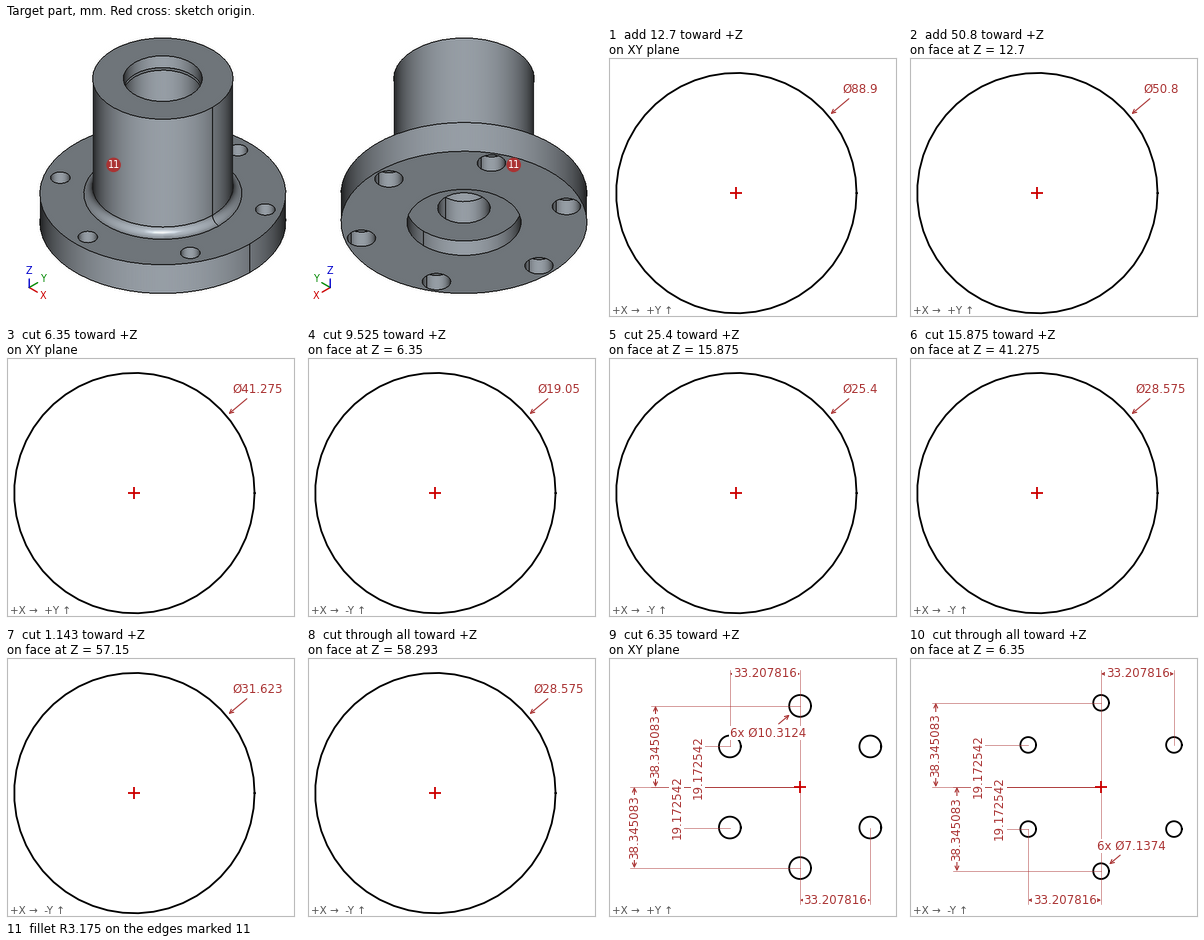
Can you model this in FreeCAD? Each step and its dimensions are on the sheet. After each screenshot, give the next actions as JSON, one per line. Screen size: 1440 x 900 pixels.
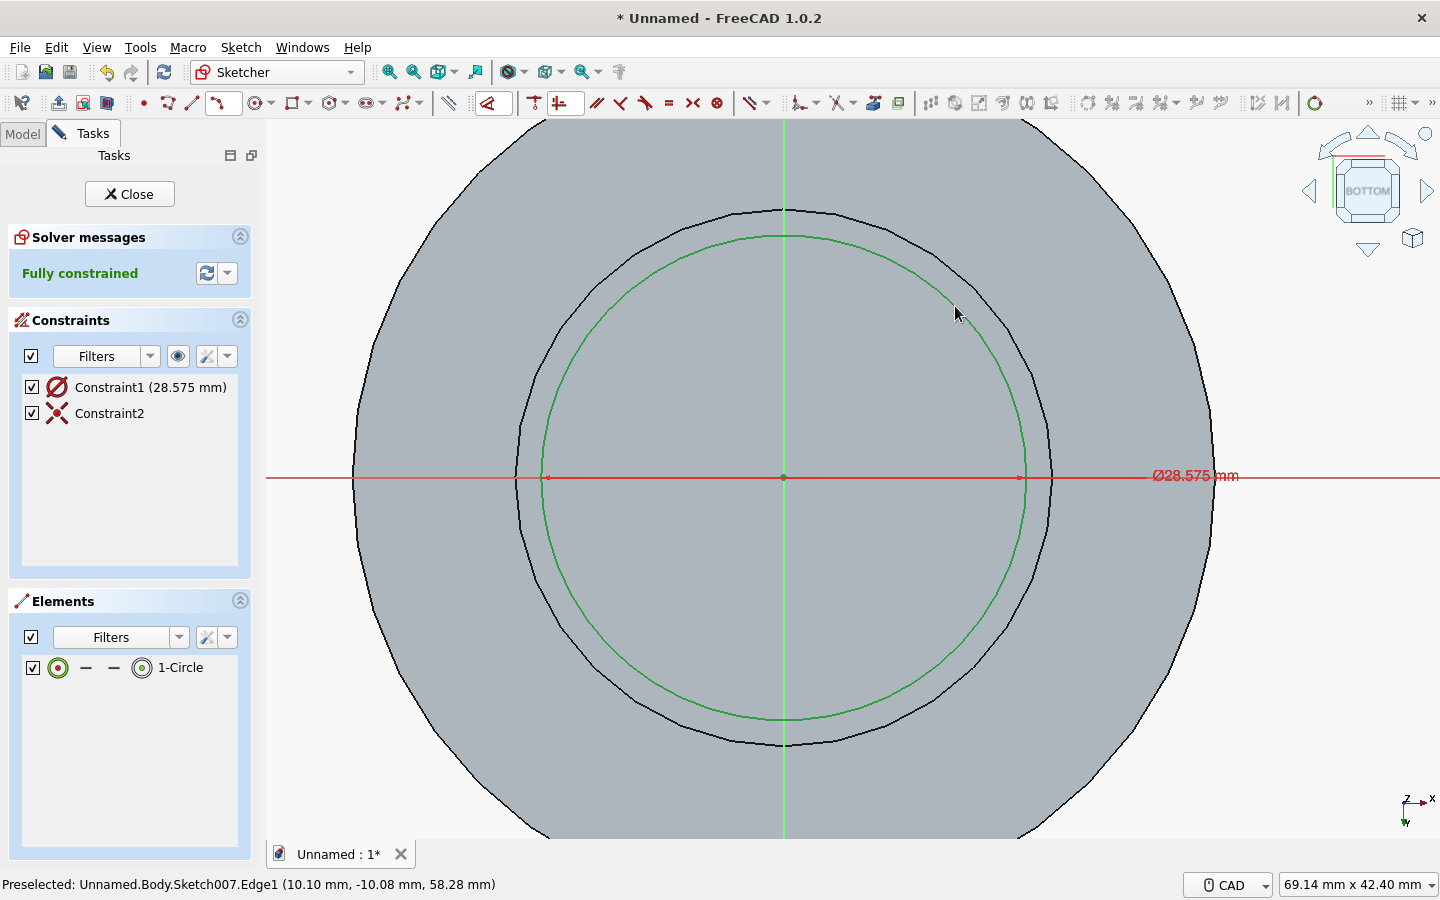
{"action": "left_click", "coordinate": [130, 194]}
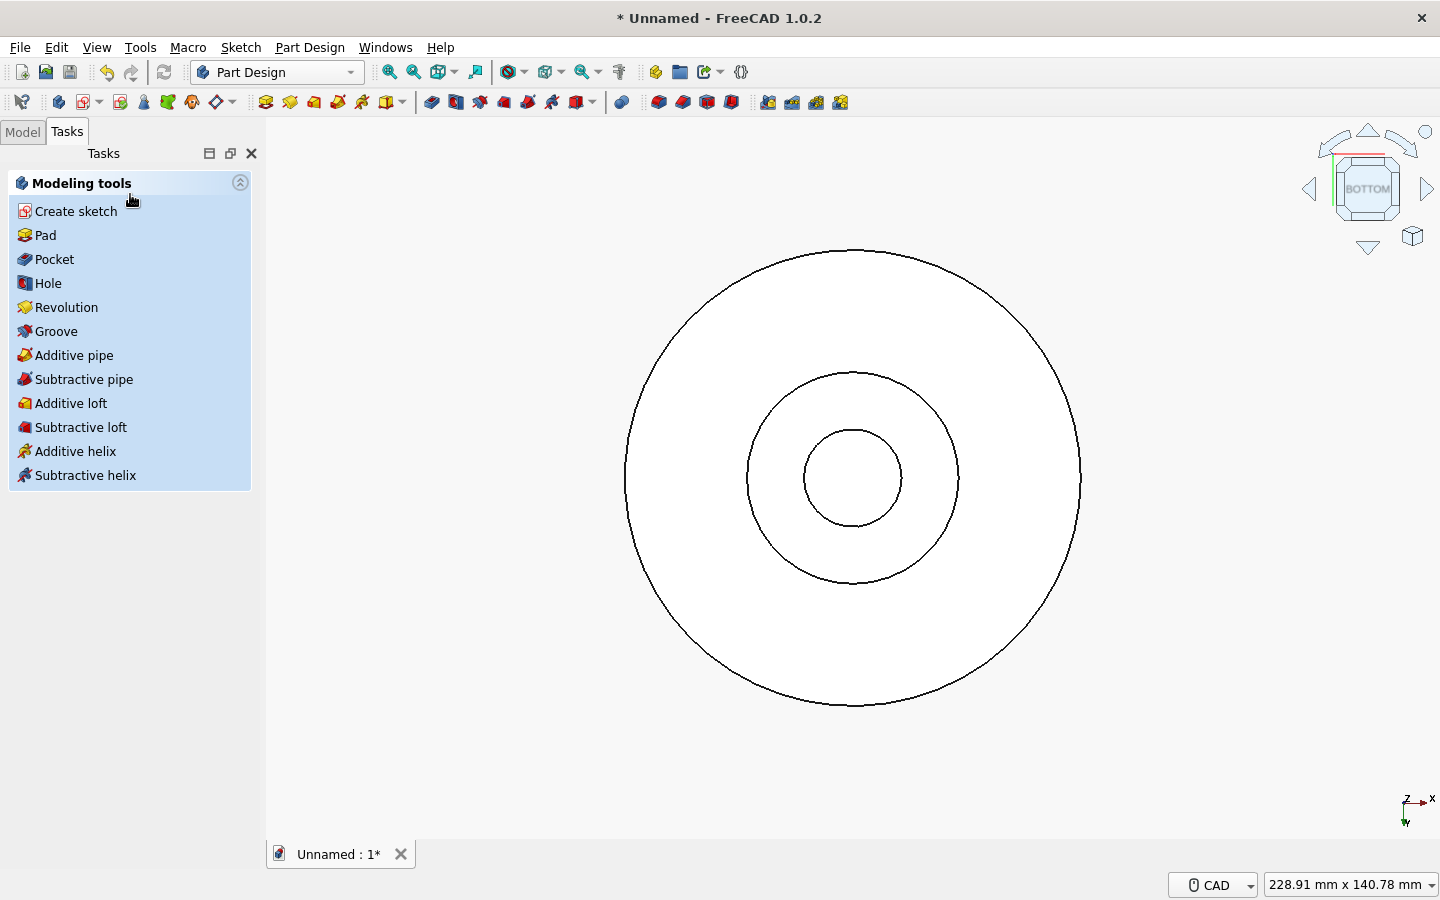
{"action": "left_click", "coordinate": [432, 102]}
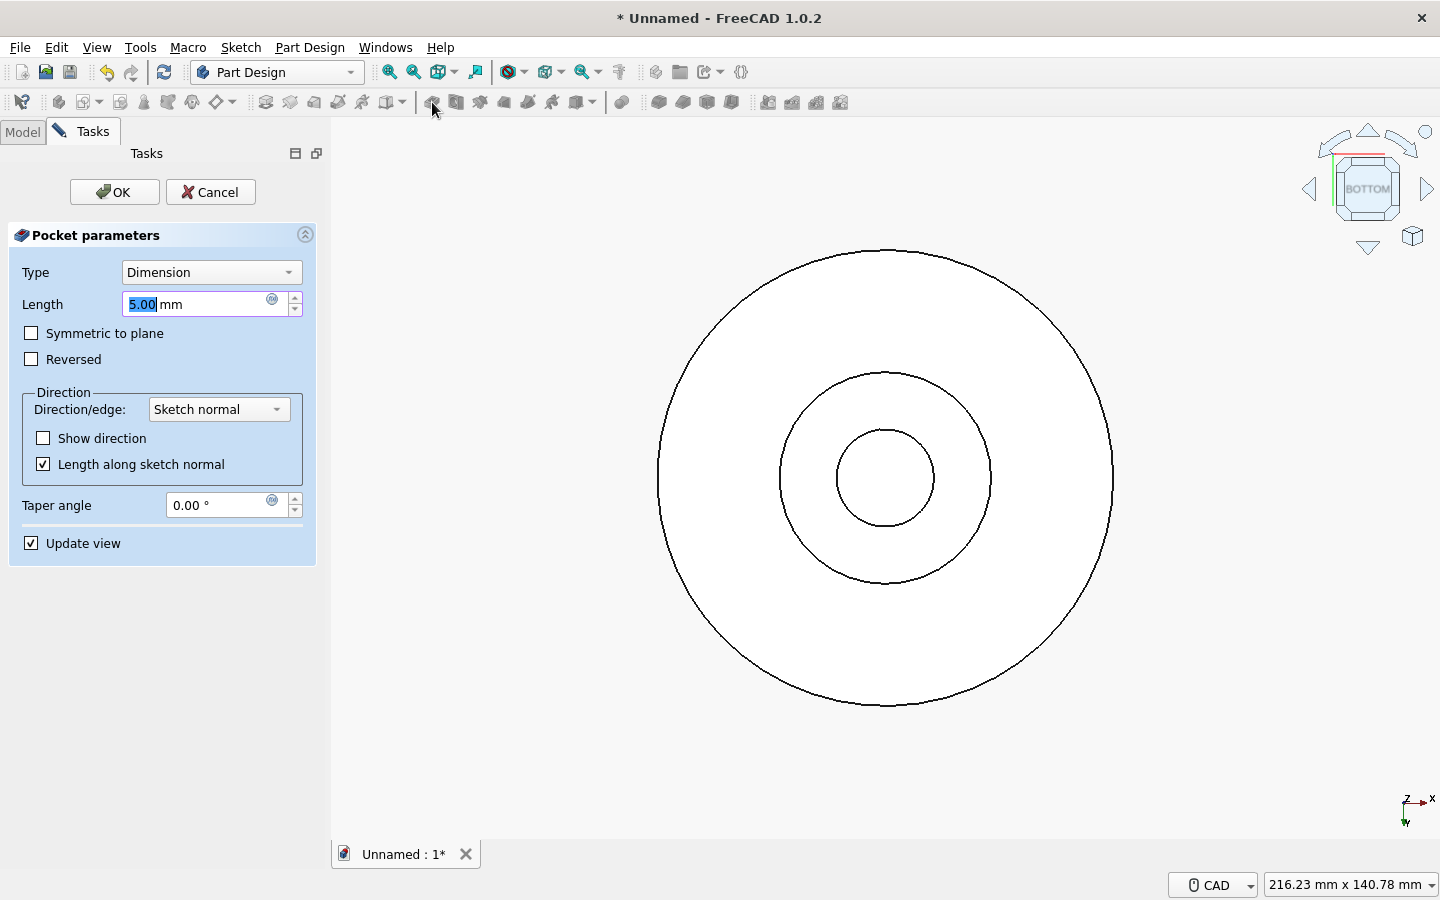
{"action": "left_click", "coordinate": [212, 272]}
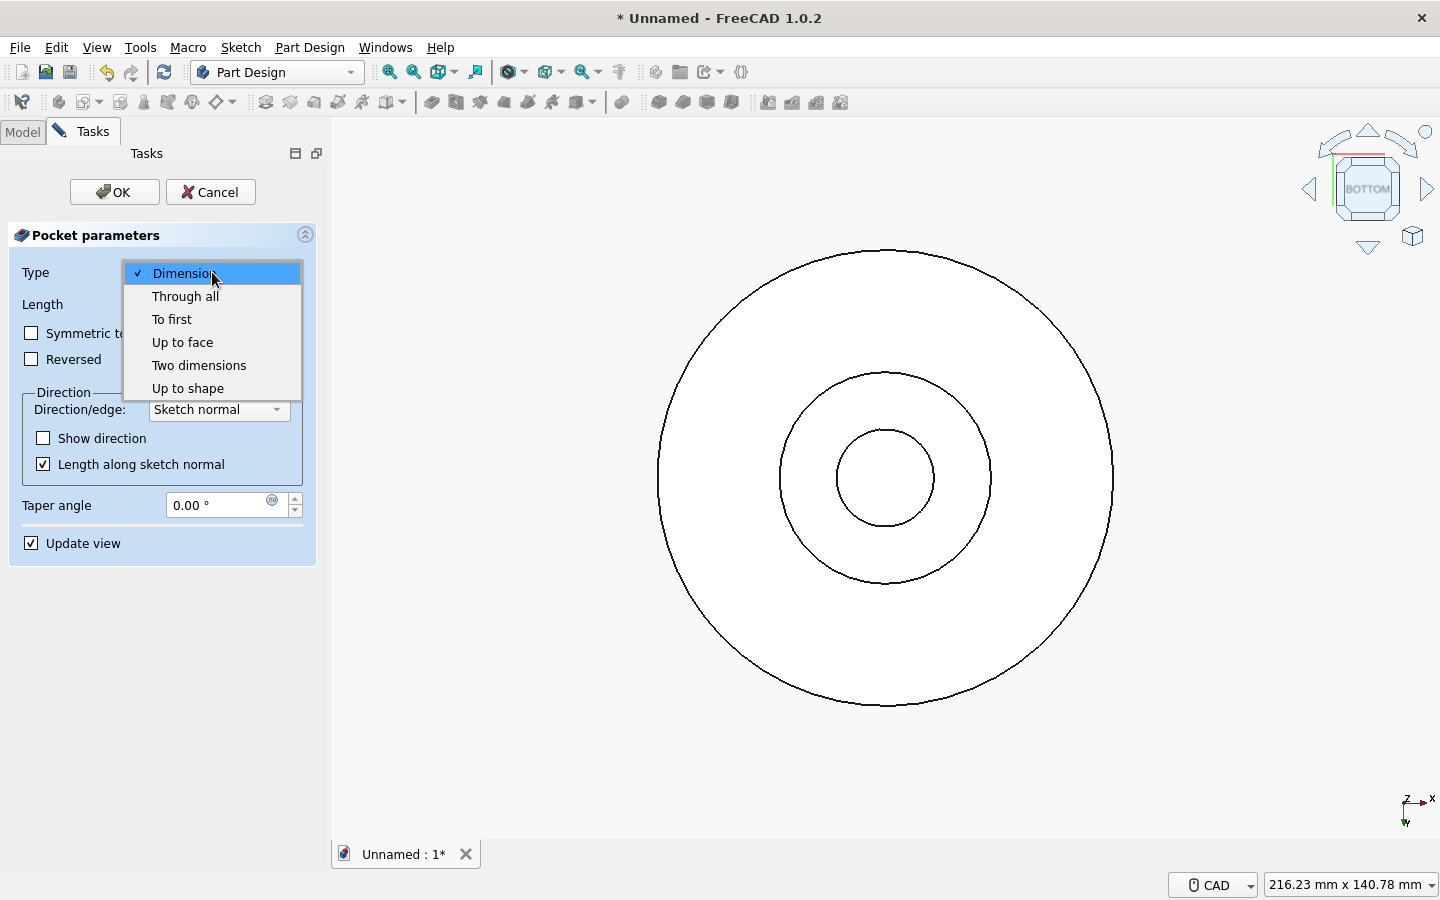
{"action": "left_click", "coordinate": [212, 296]}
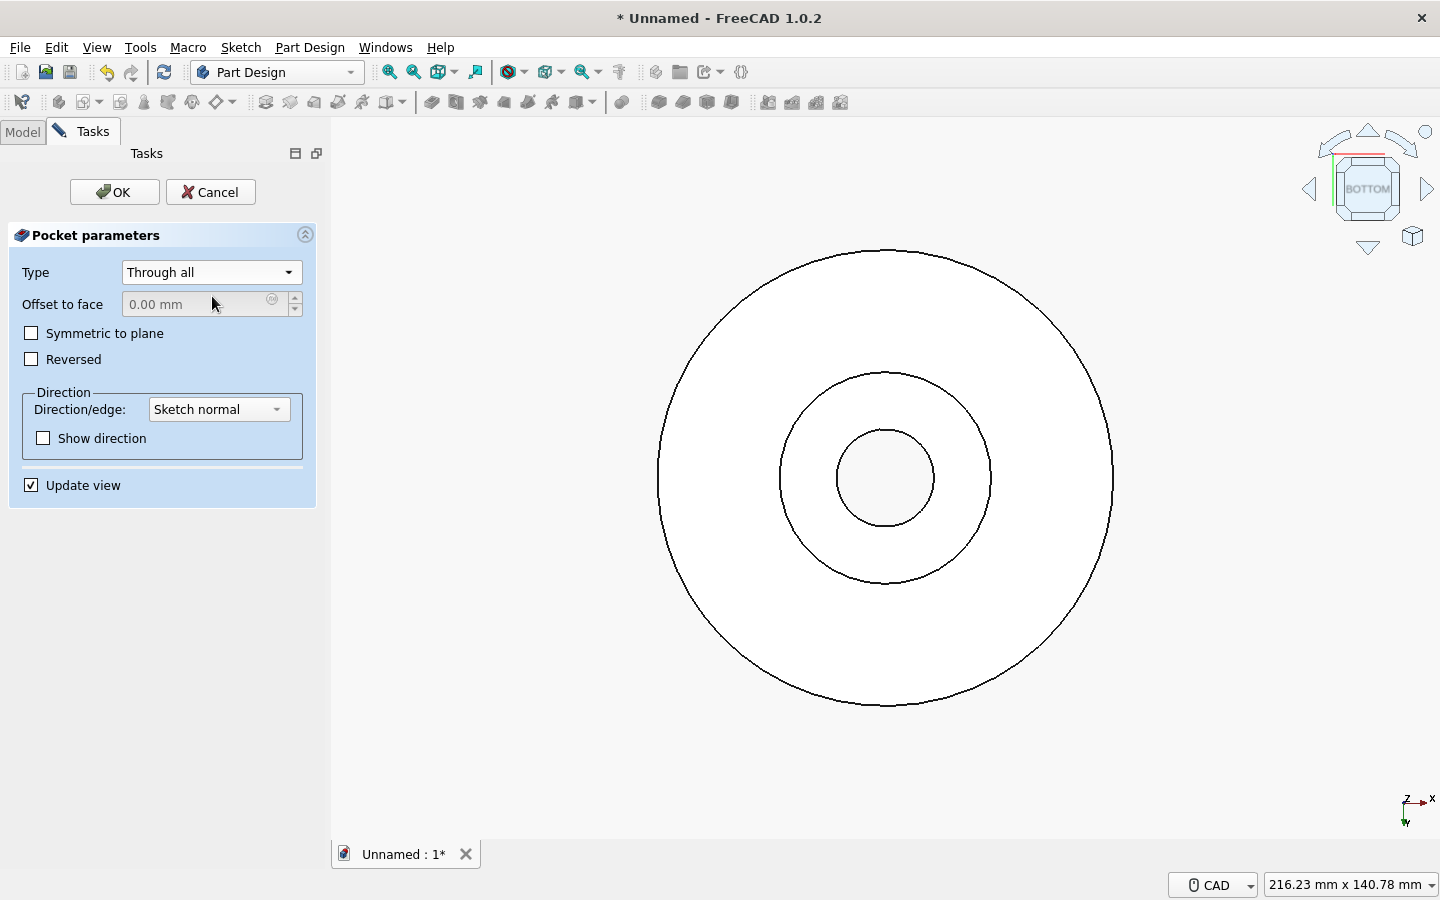
{"action": "left_click", "coordinate": [115, 192]}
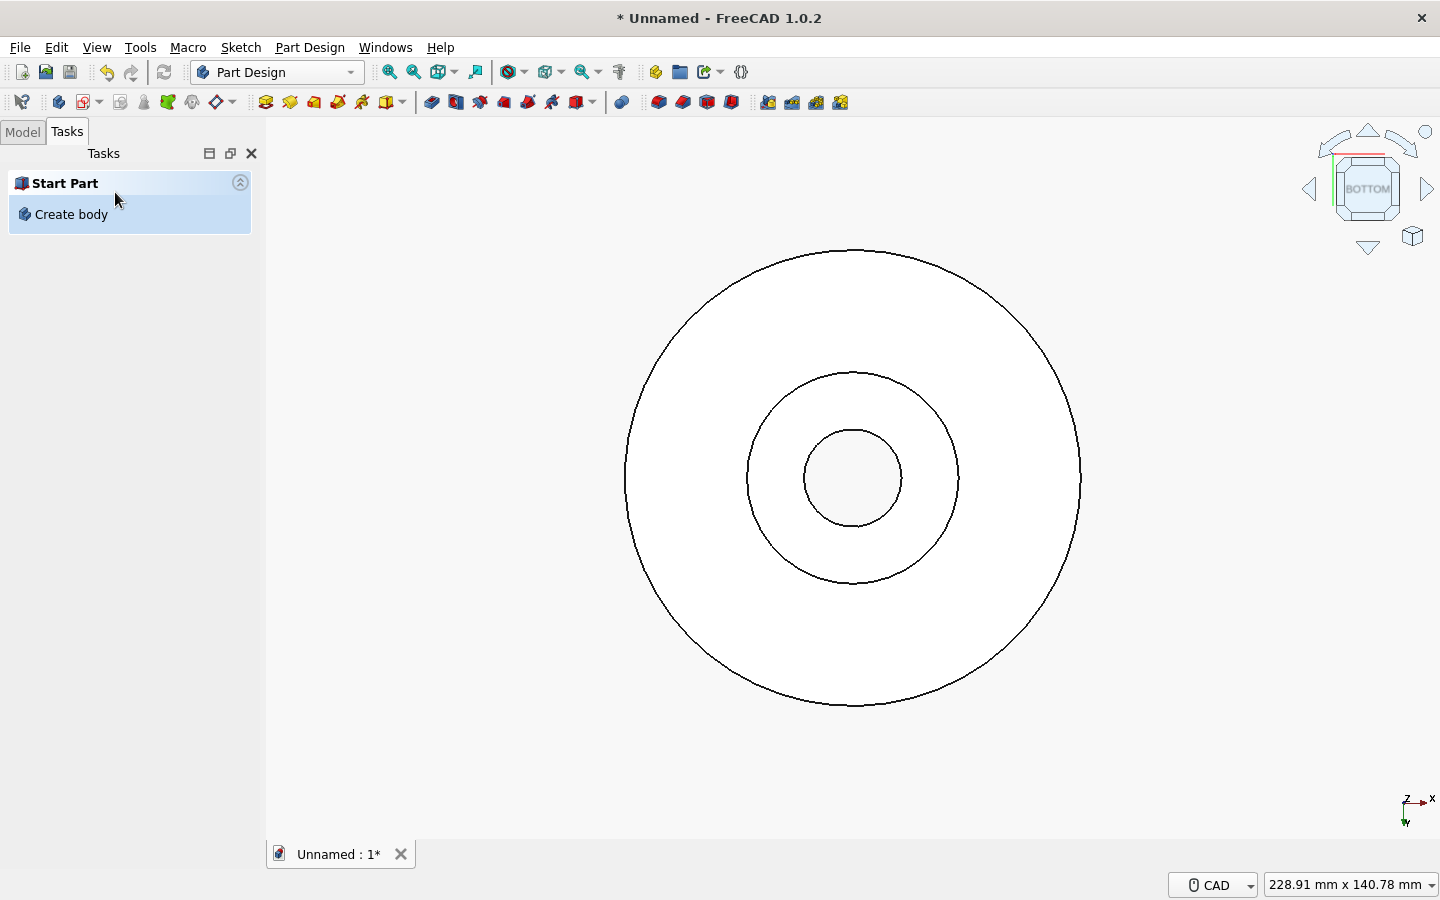
{"action": "left_click", "coordinate": [84, 102]}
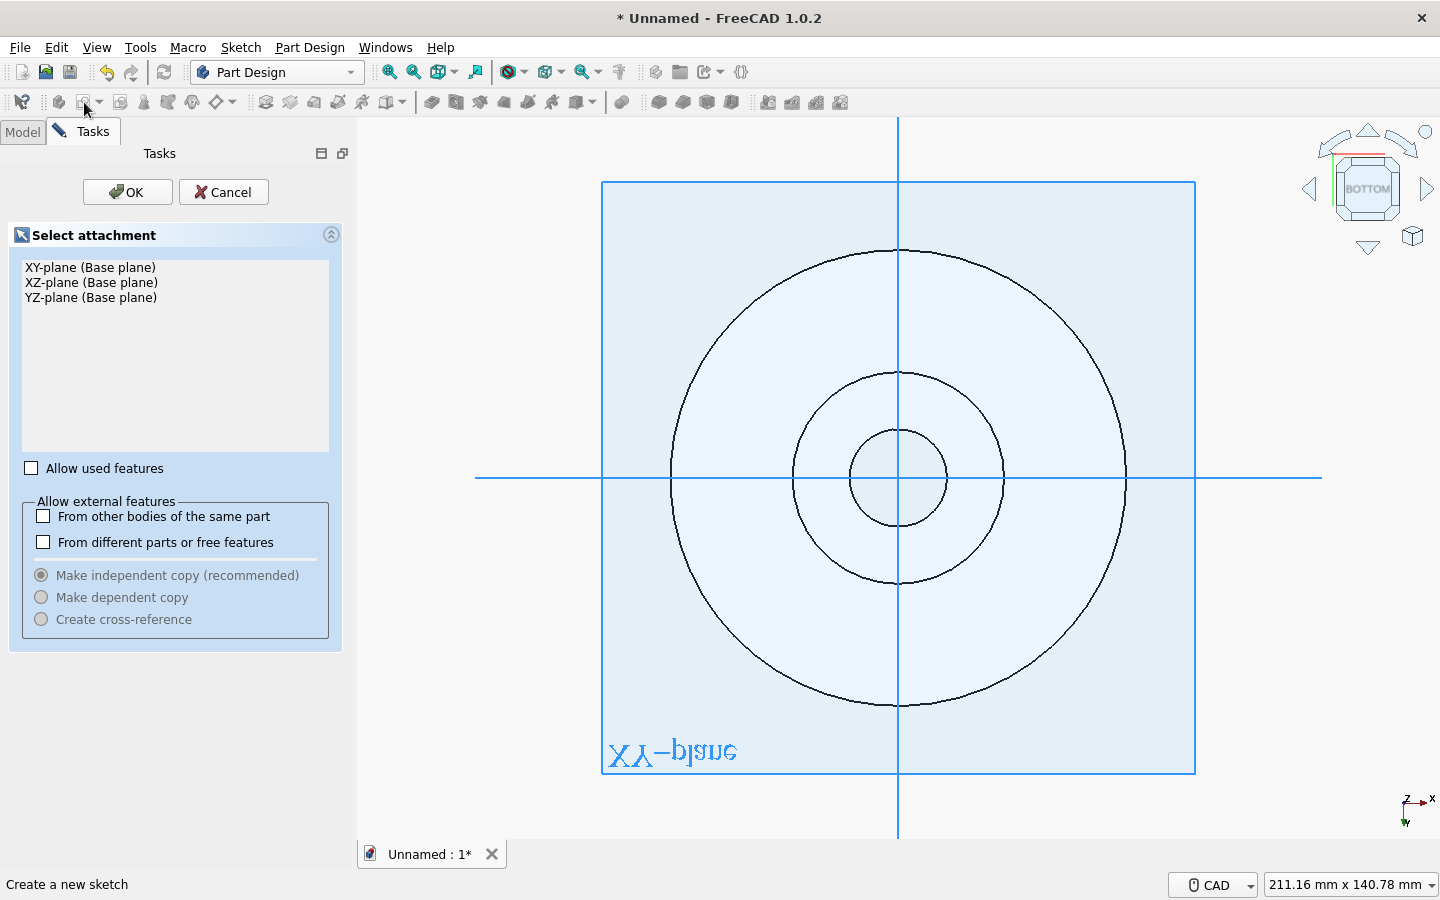
{"action": "left_click", "coordinate": [82, 268]}